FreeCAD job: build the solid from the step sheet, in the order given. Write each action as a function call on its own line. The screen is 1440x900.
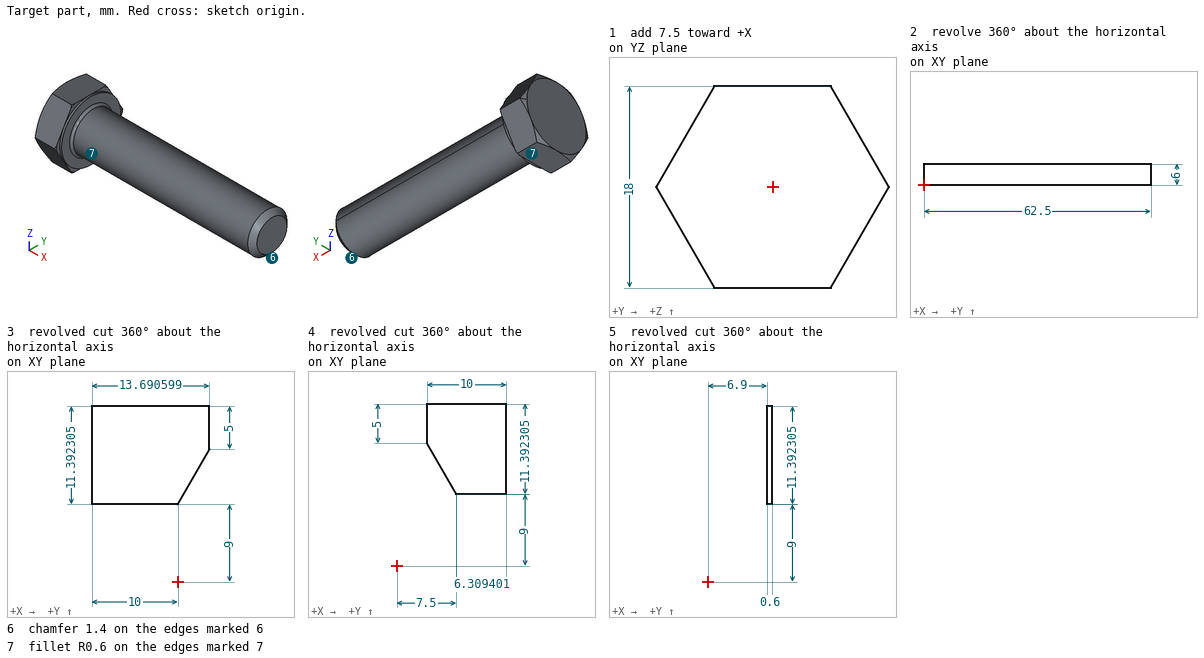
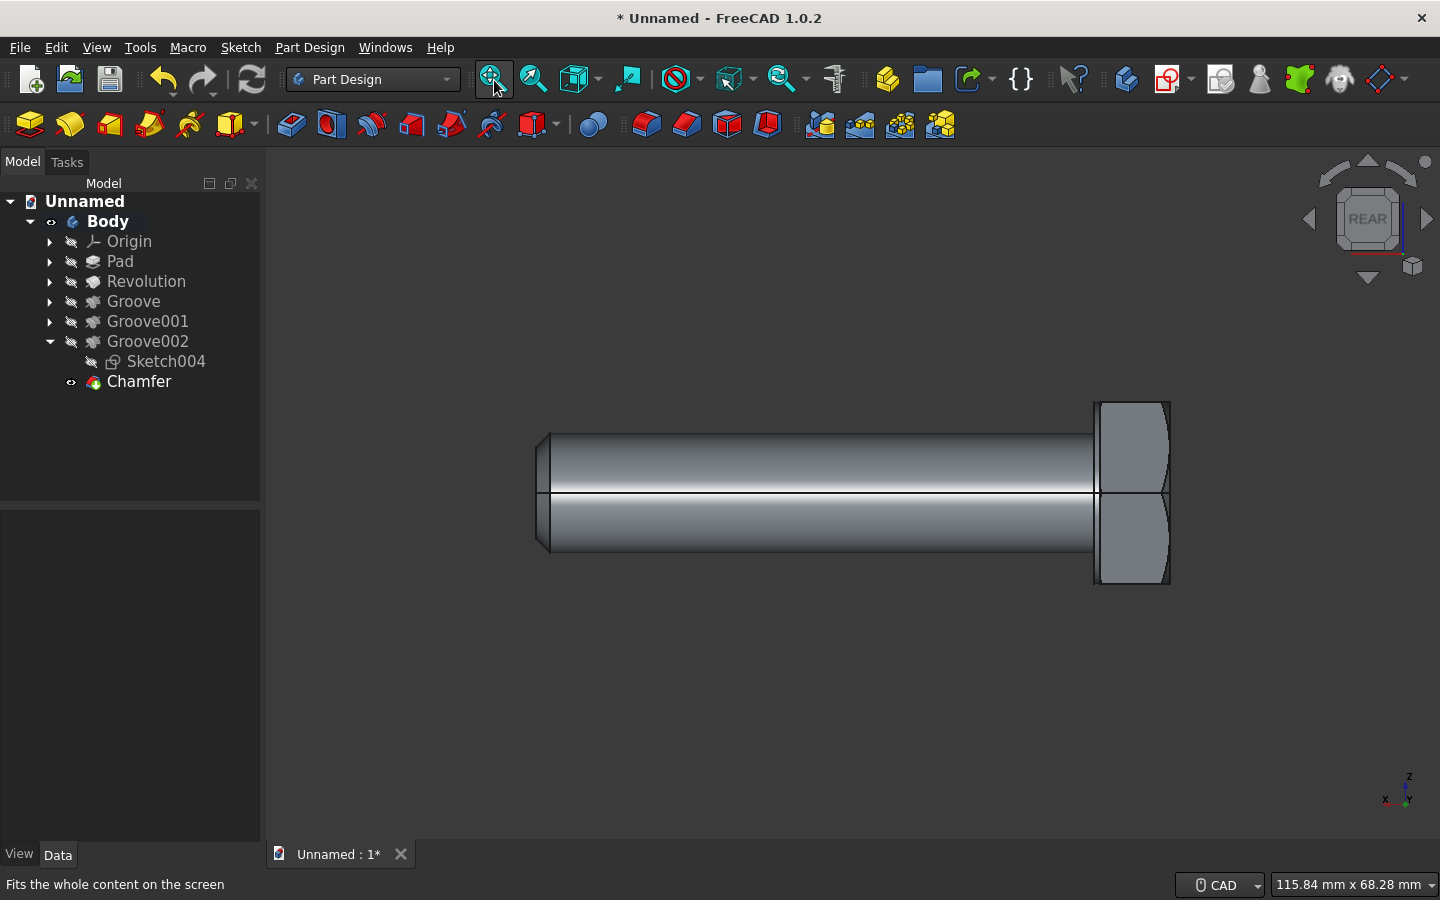
key(6)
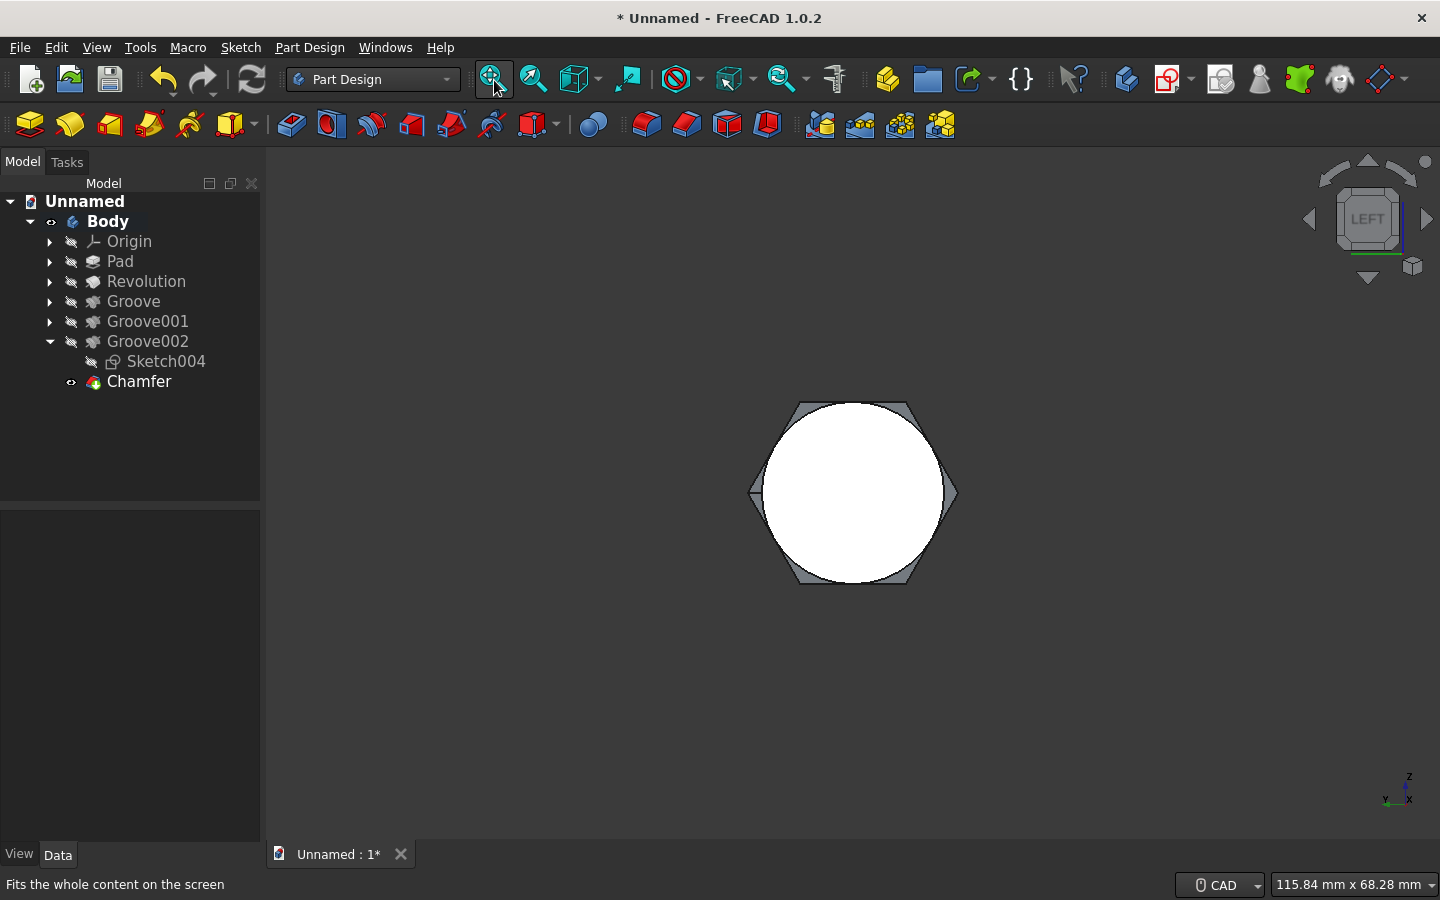
click(494, 80)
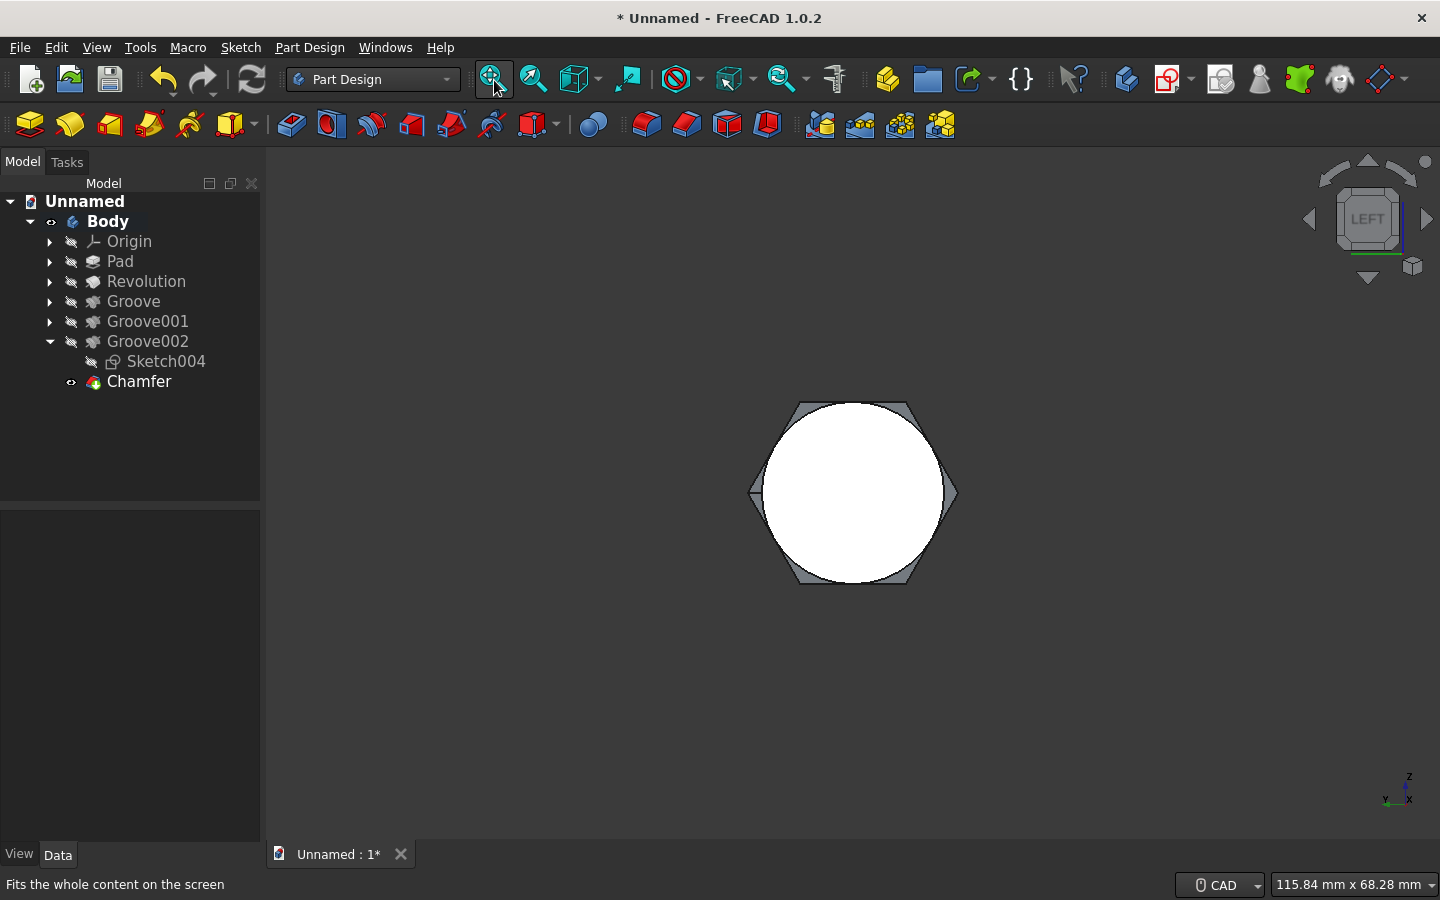
key(v)
key(3)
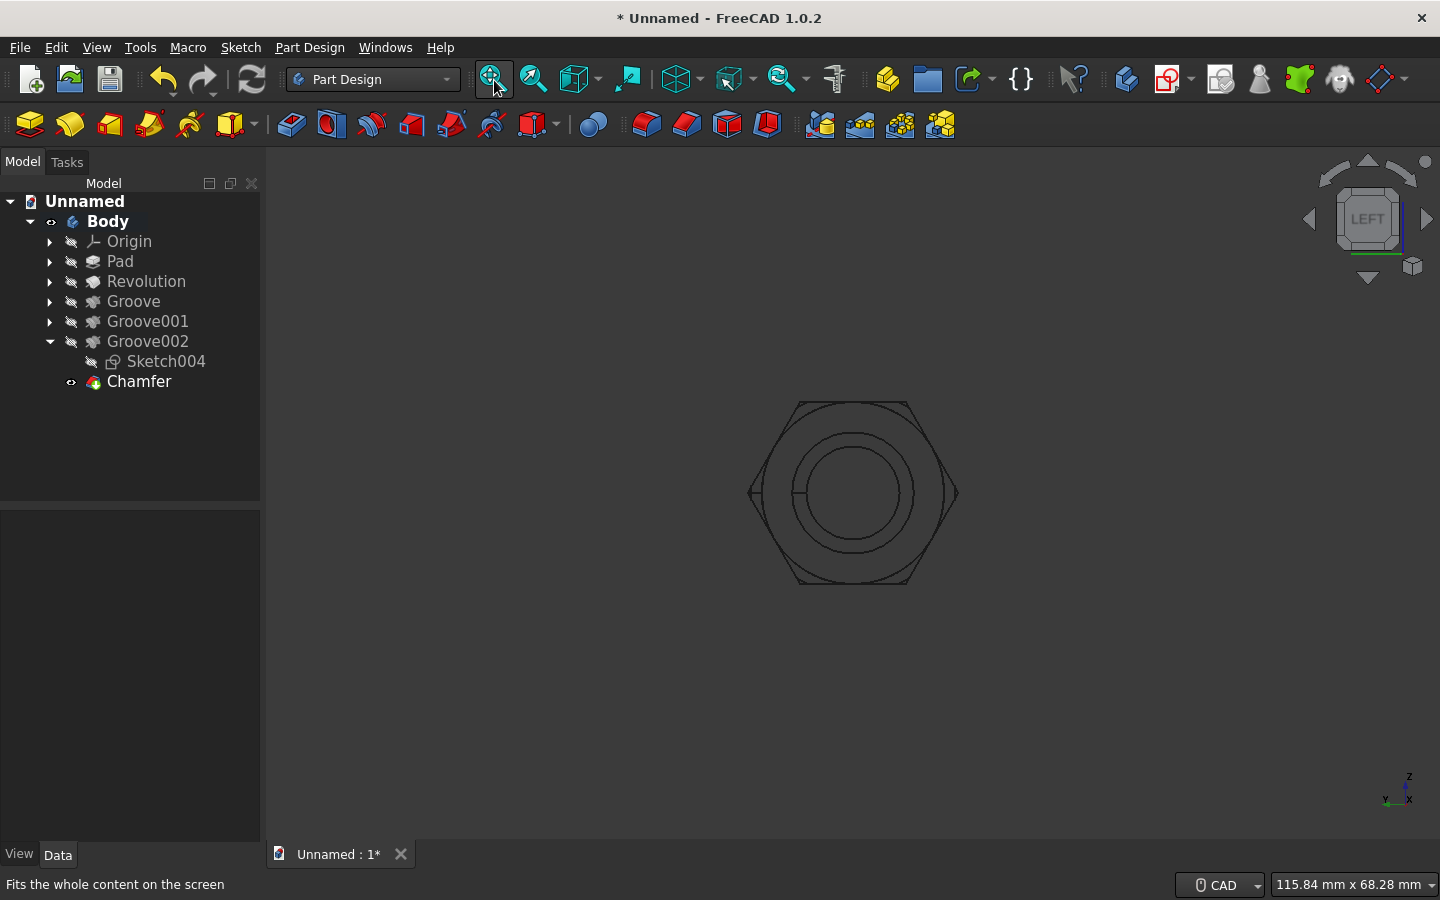
key(0)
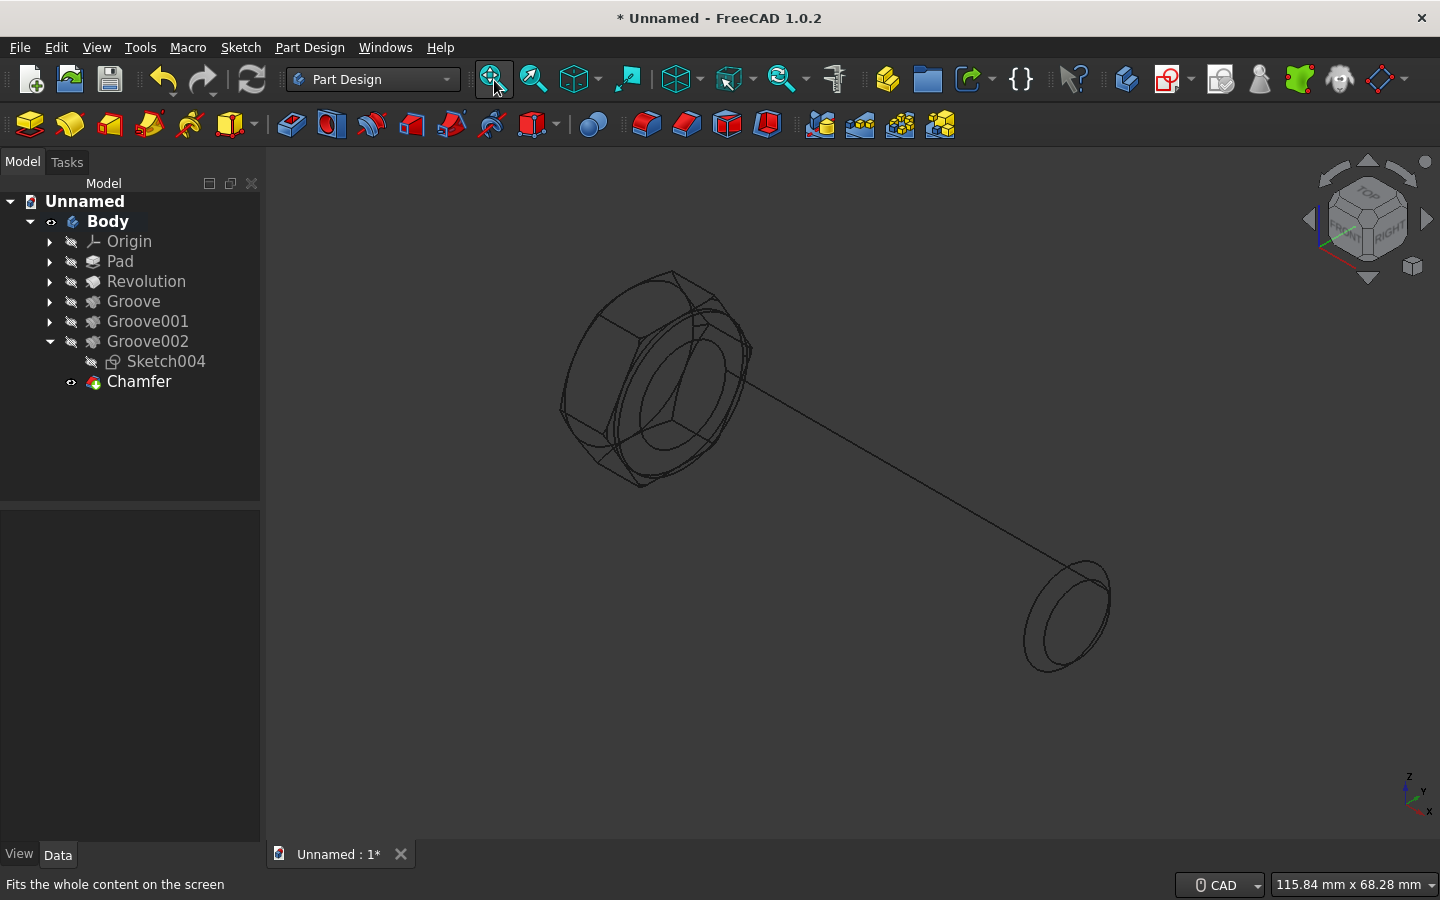
click(640, 419)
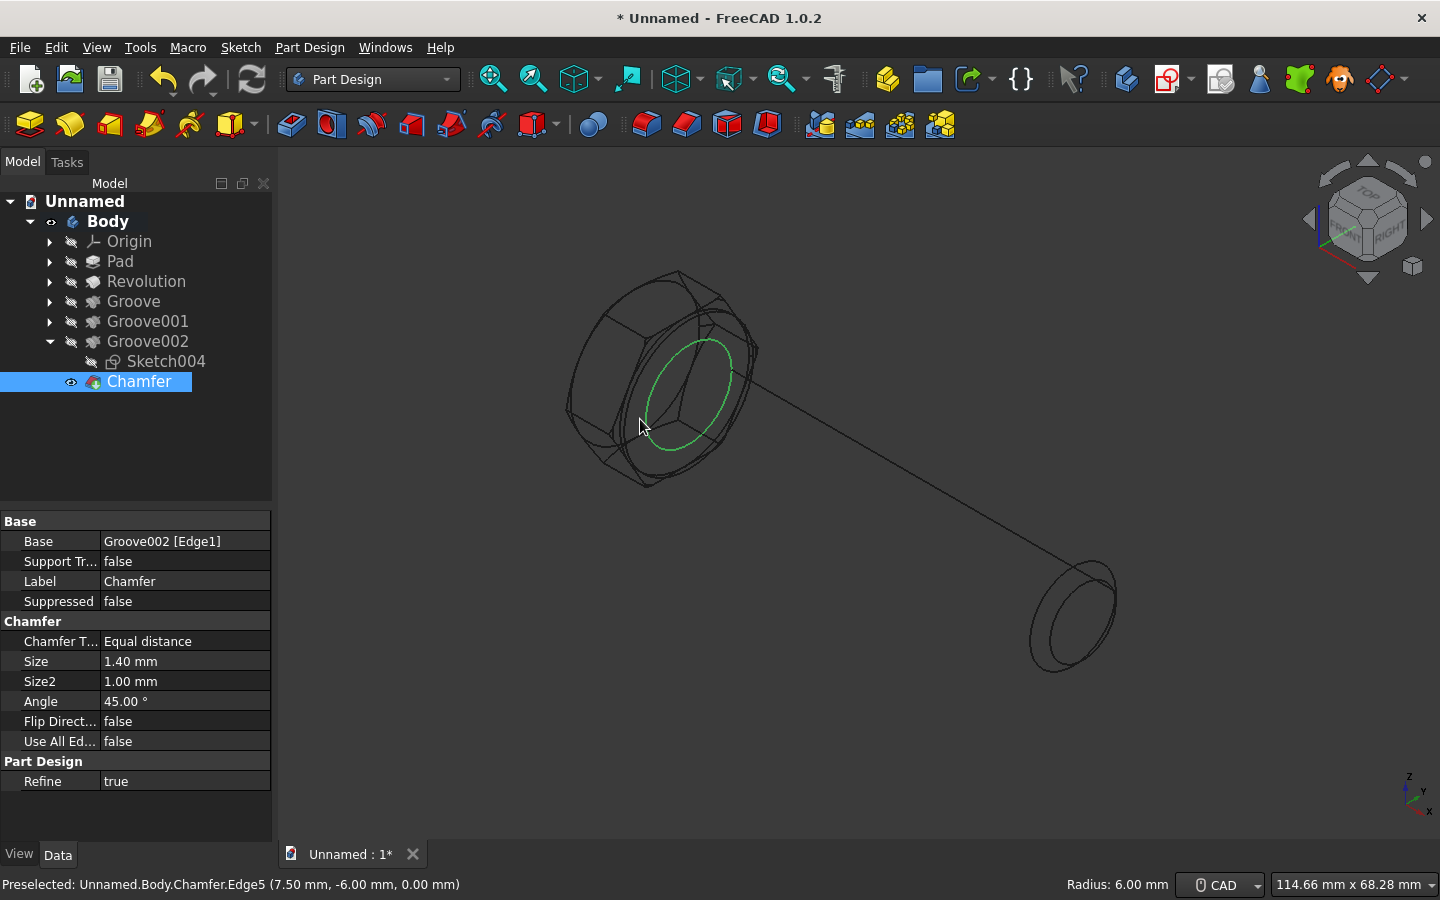
key(v)
key(1)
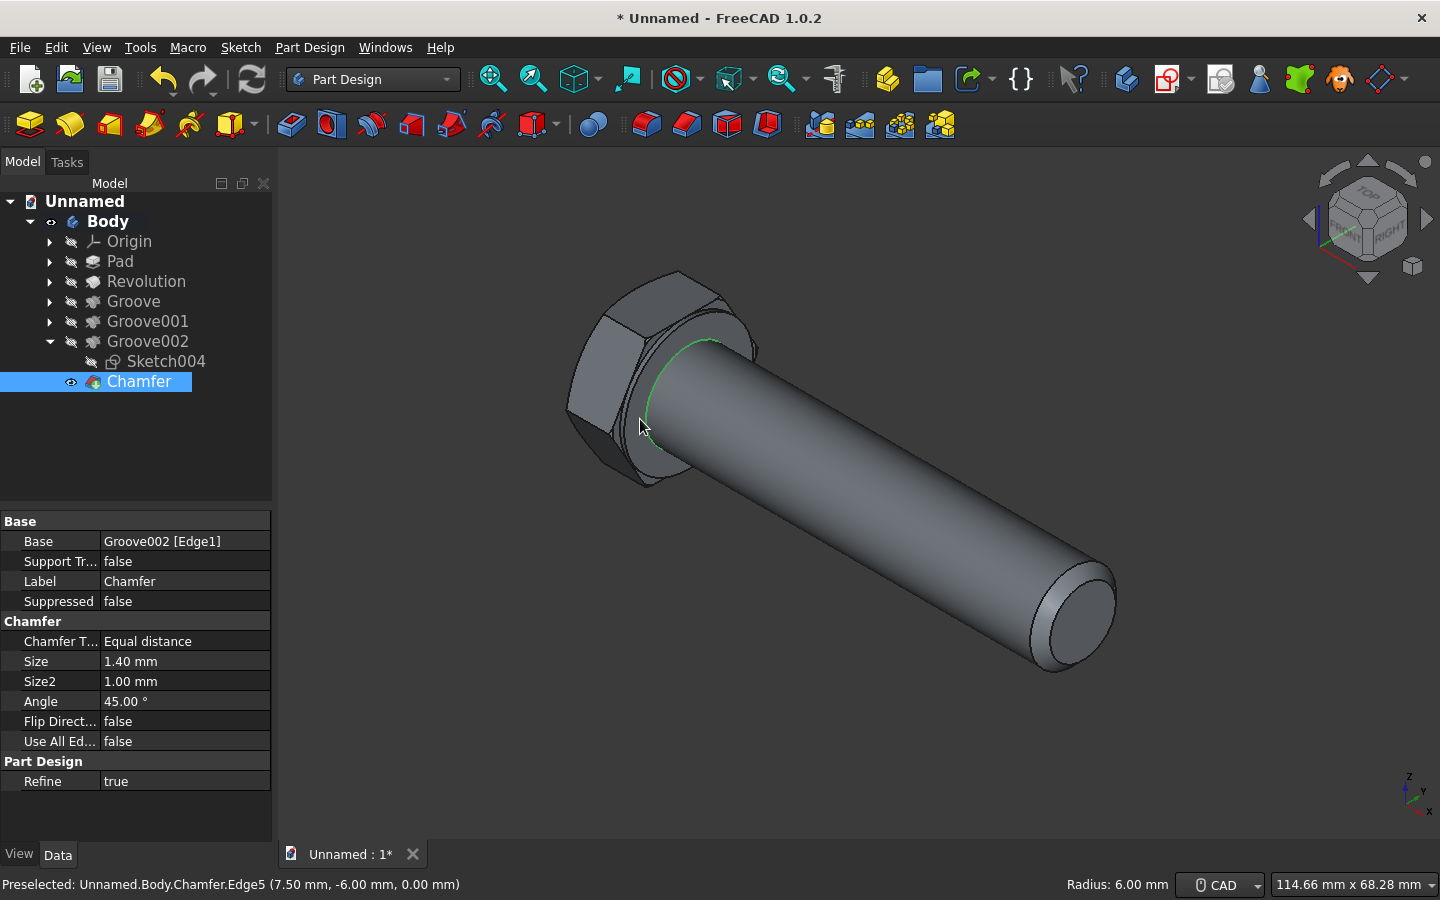
click(648, 124)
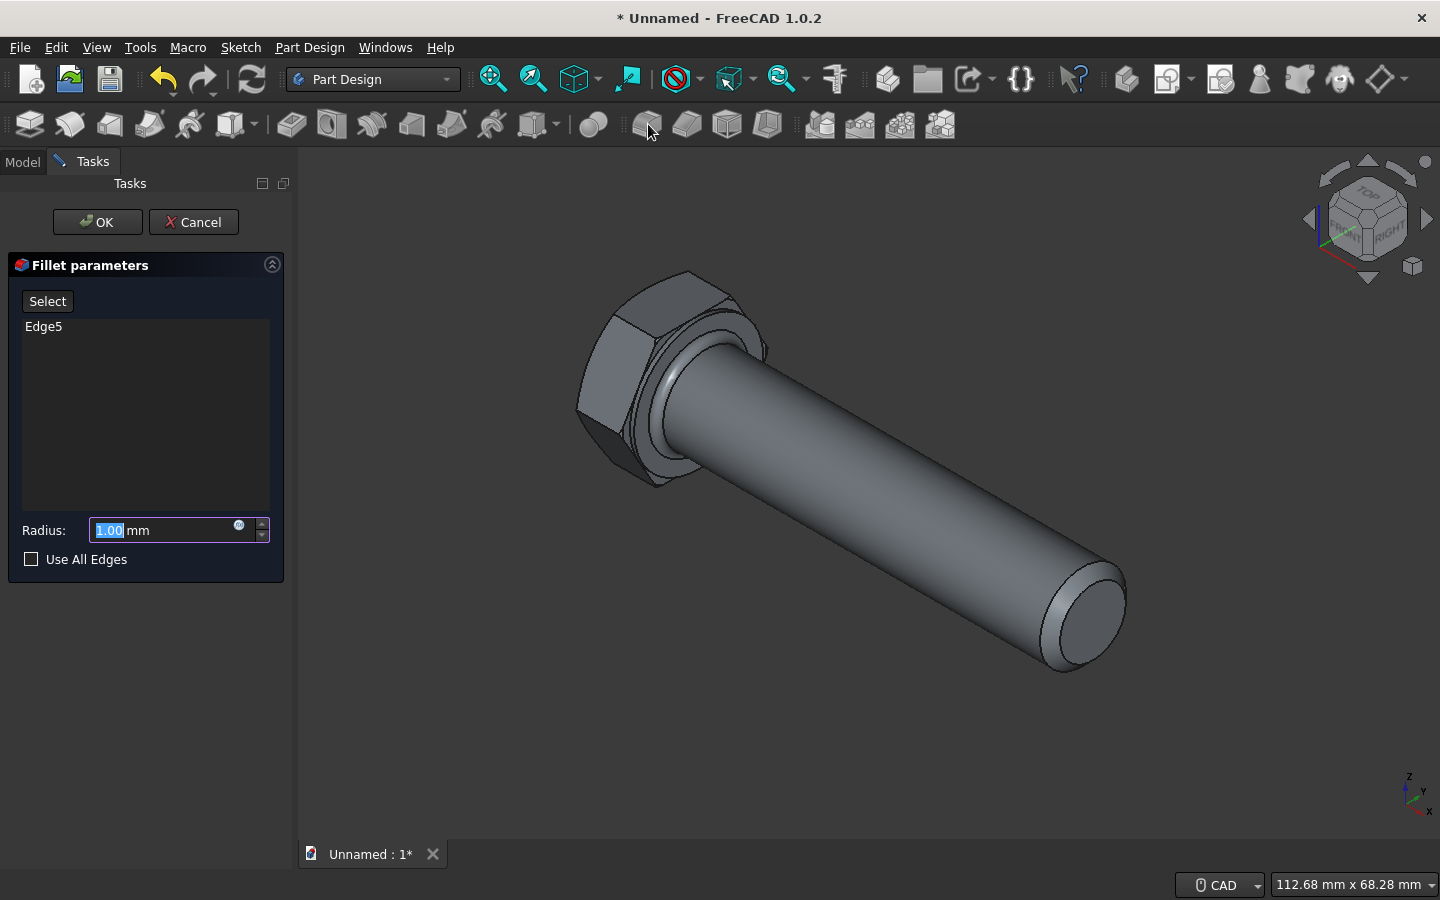
text(0.6)
key(Tab)